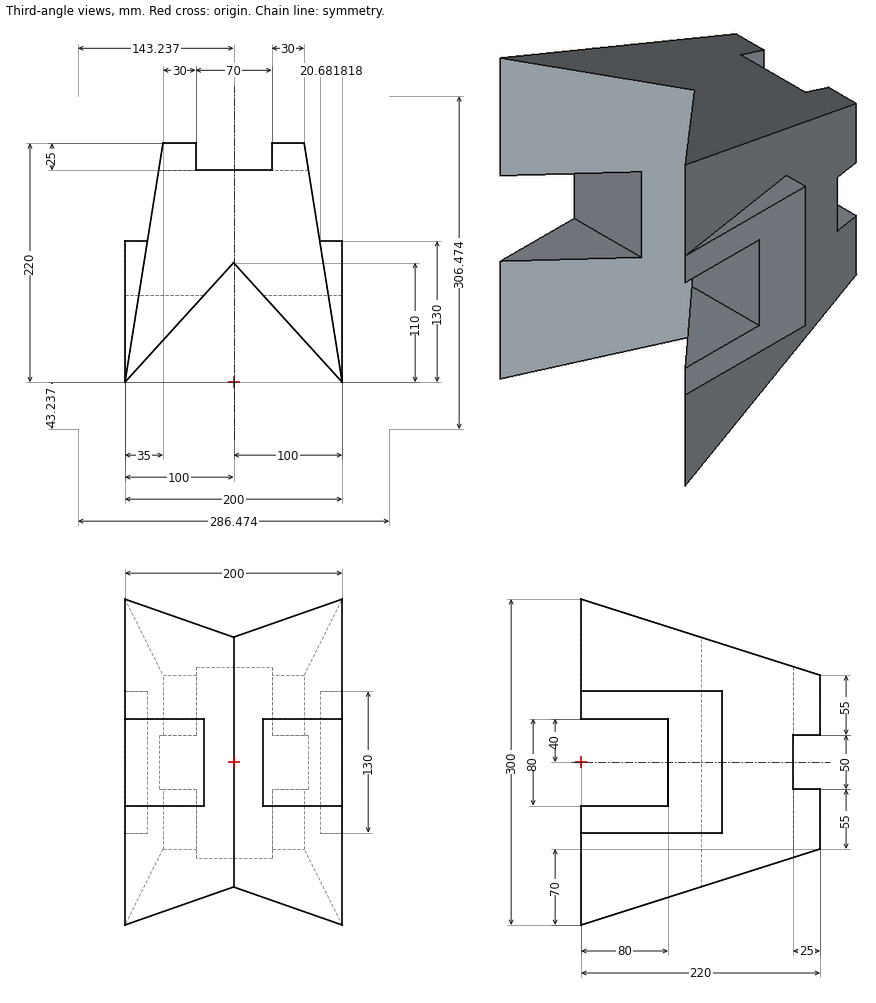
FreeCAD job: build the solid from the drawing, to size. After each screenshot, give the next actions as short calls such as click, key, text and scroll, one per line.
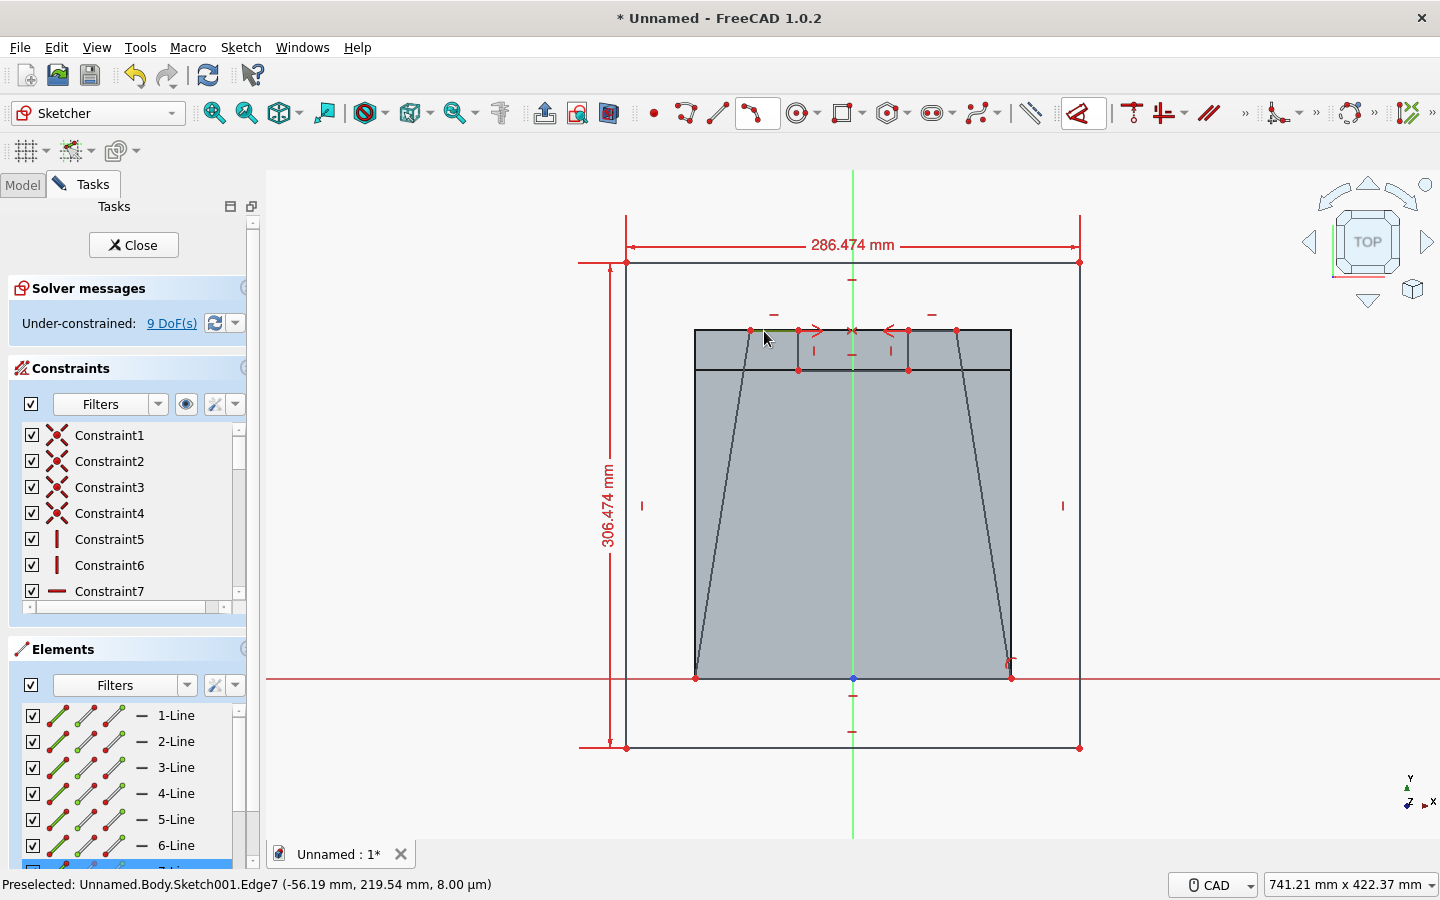
key(l)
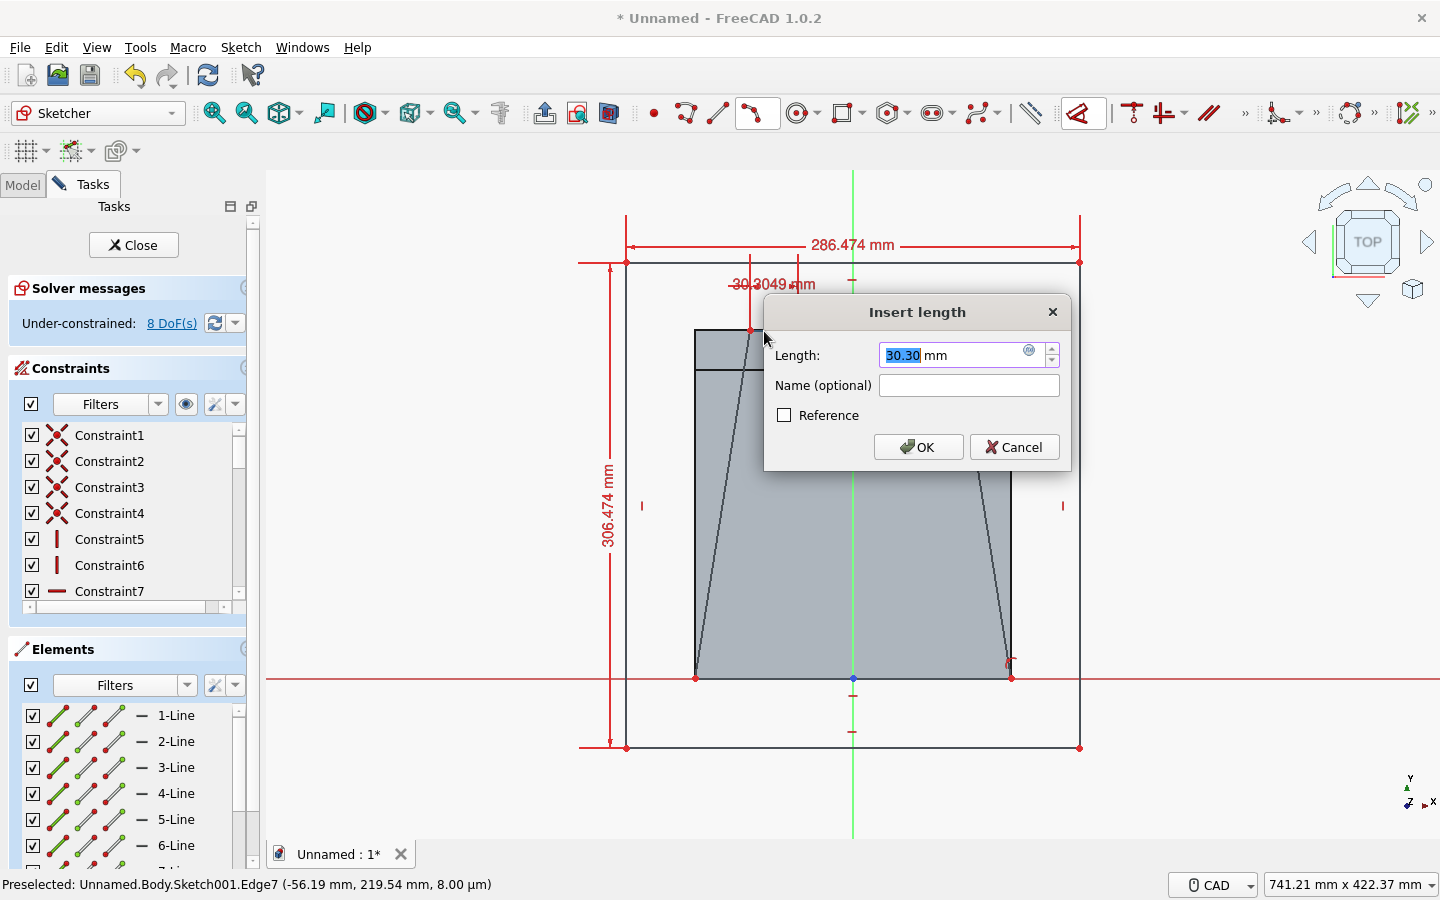
text(30)
key(Return)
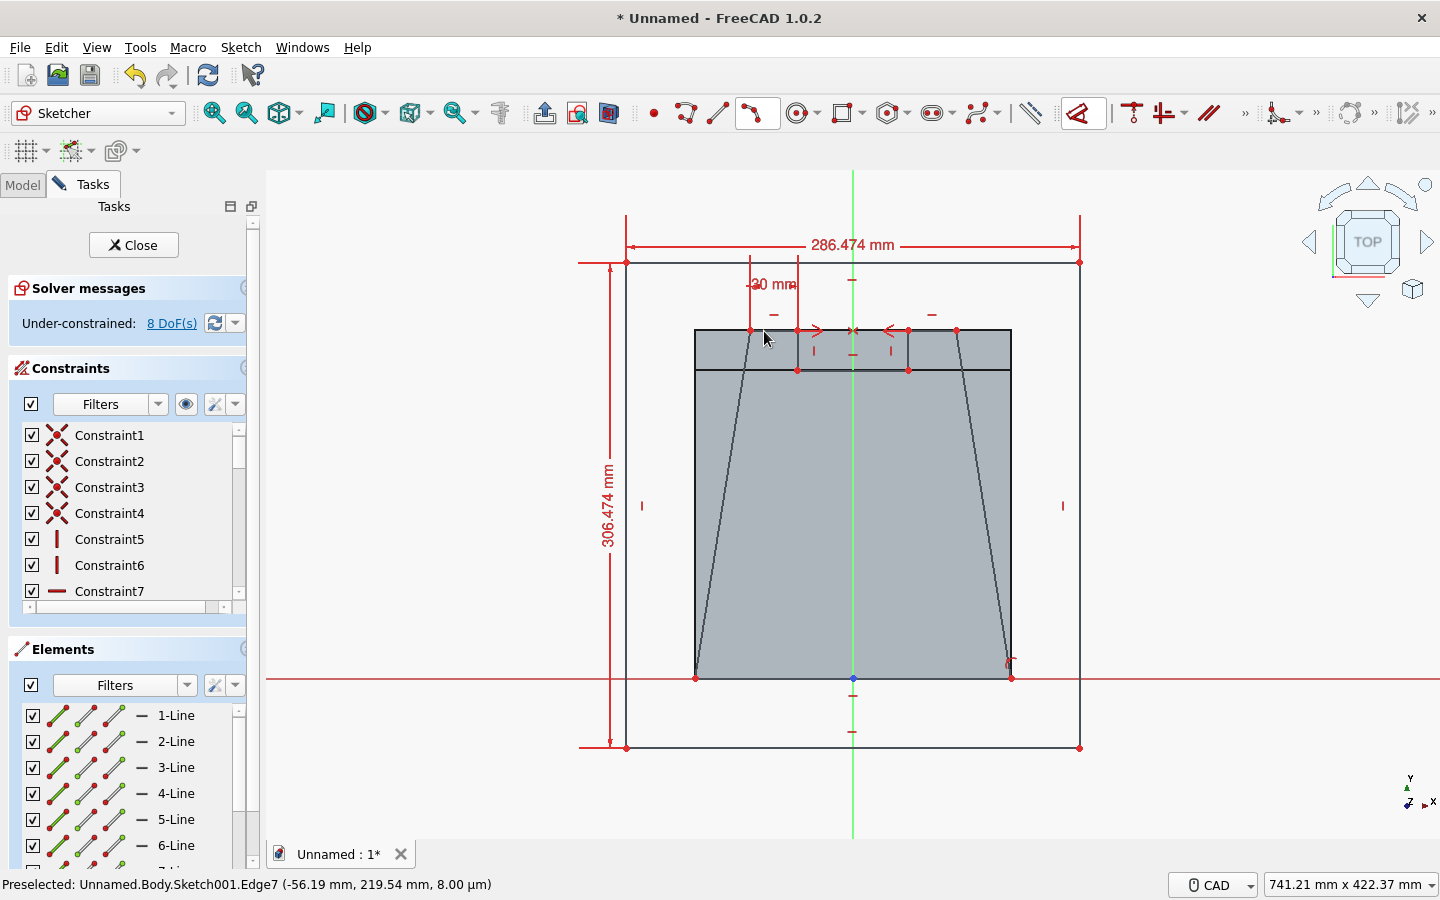
click(798, 343)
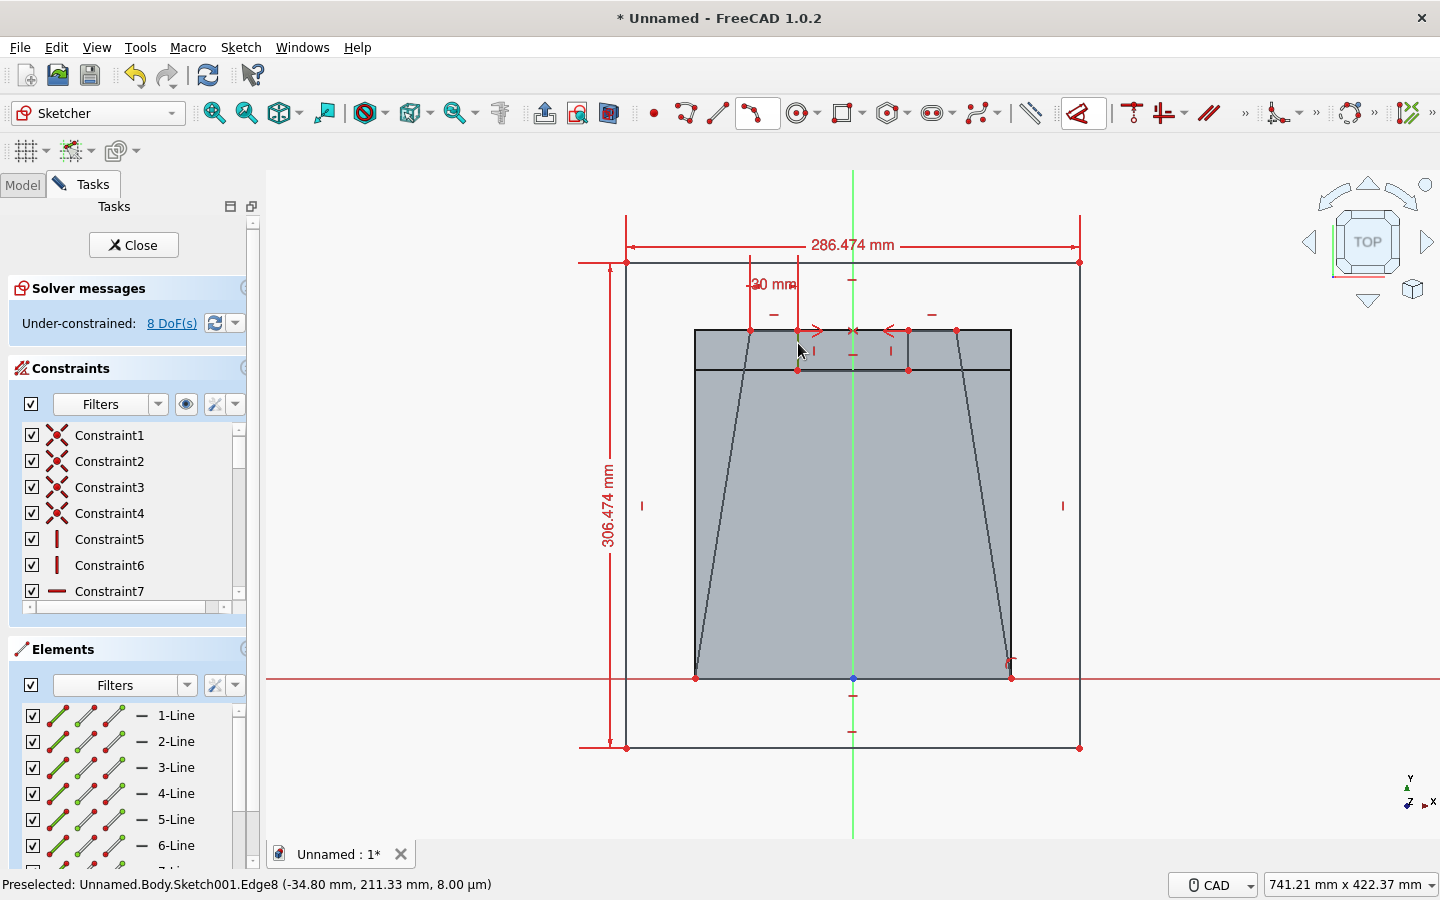
key(i)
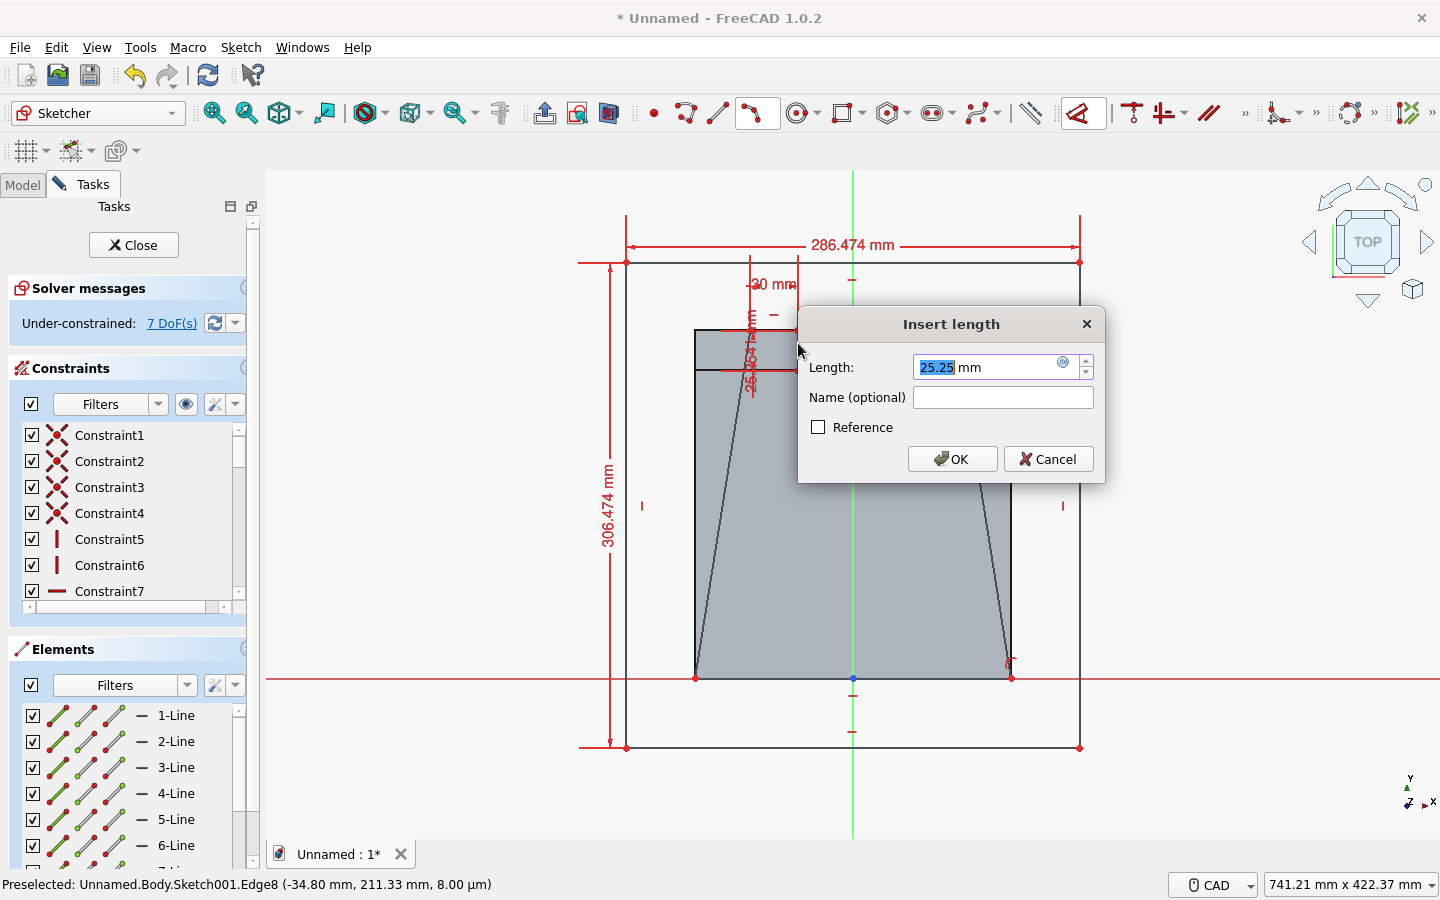
text(25)
key(Return)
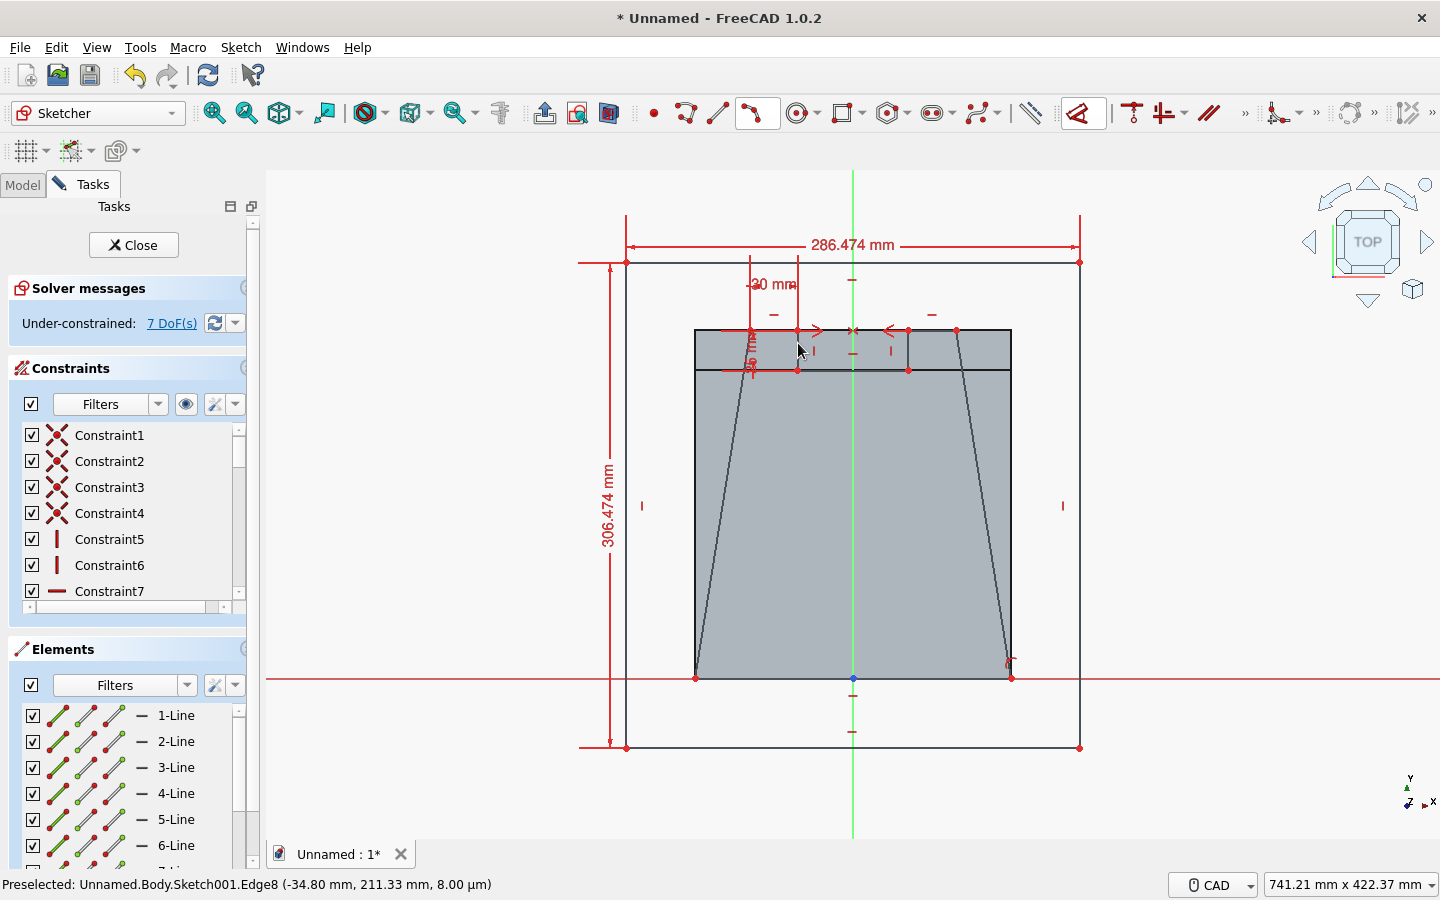
click(831, 371)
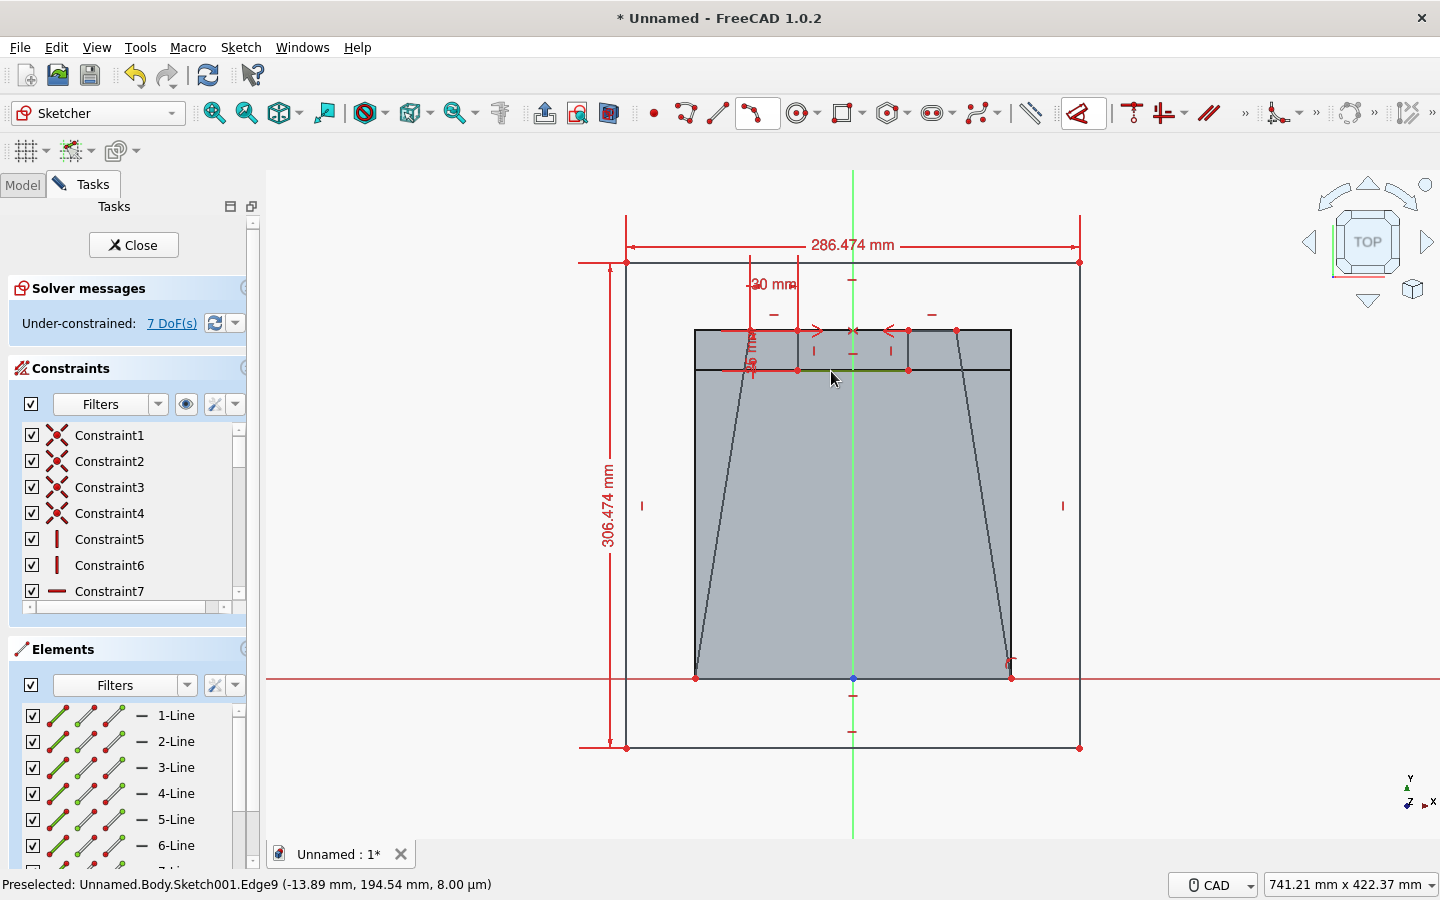
key(l)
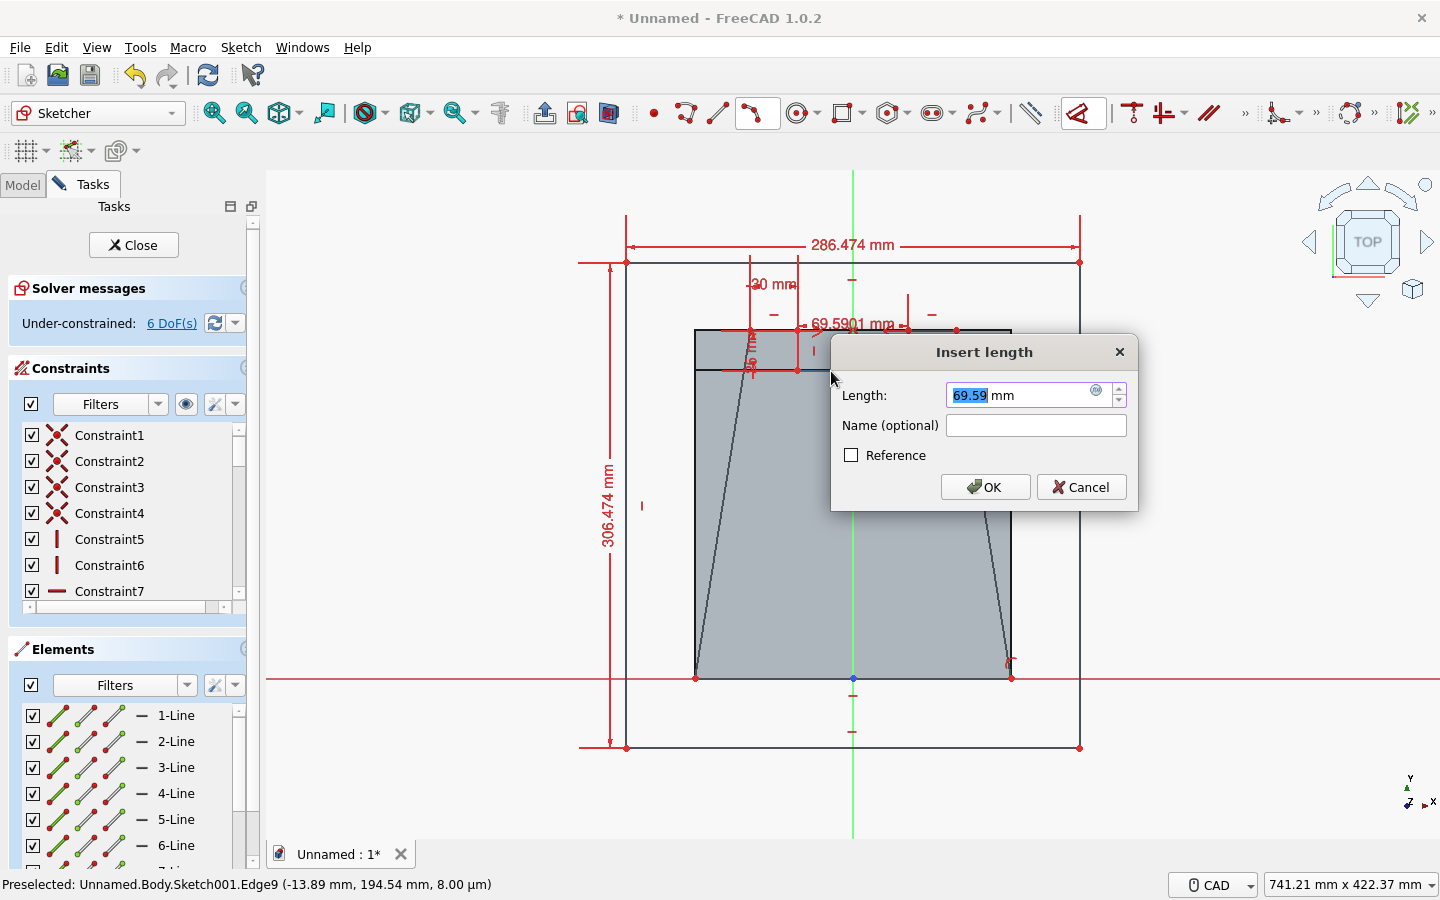
text(70)
key(Return)